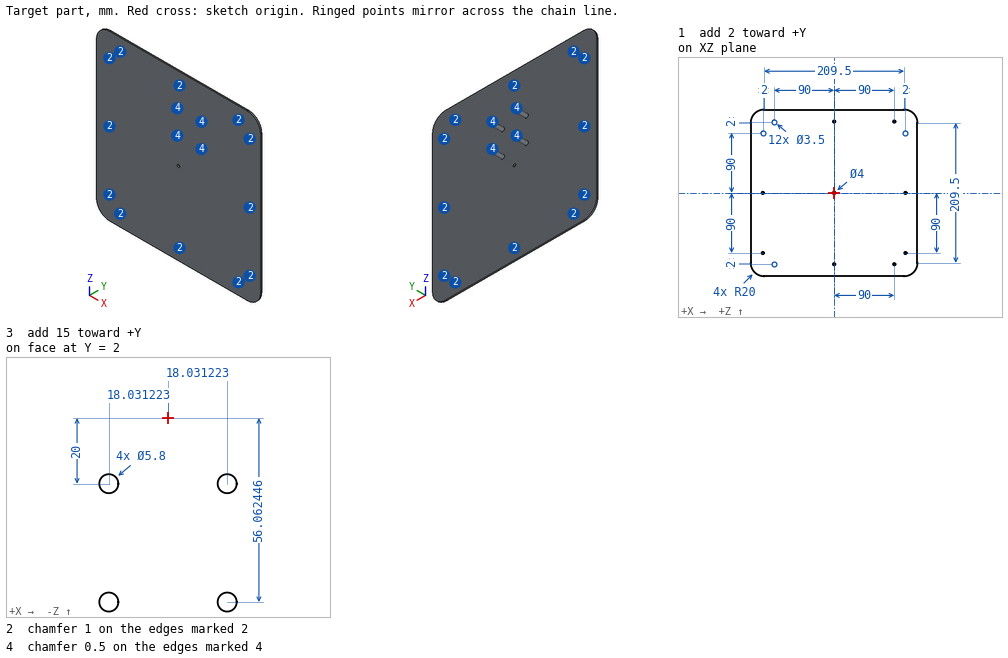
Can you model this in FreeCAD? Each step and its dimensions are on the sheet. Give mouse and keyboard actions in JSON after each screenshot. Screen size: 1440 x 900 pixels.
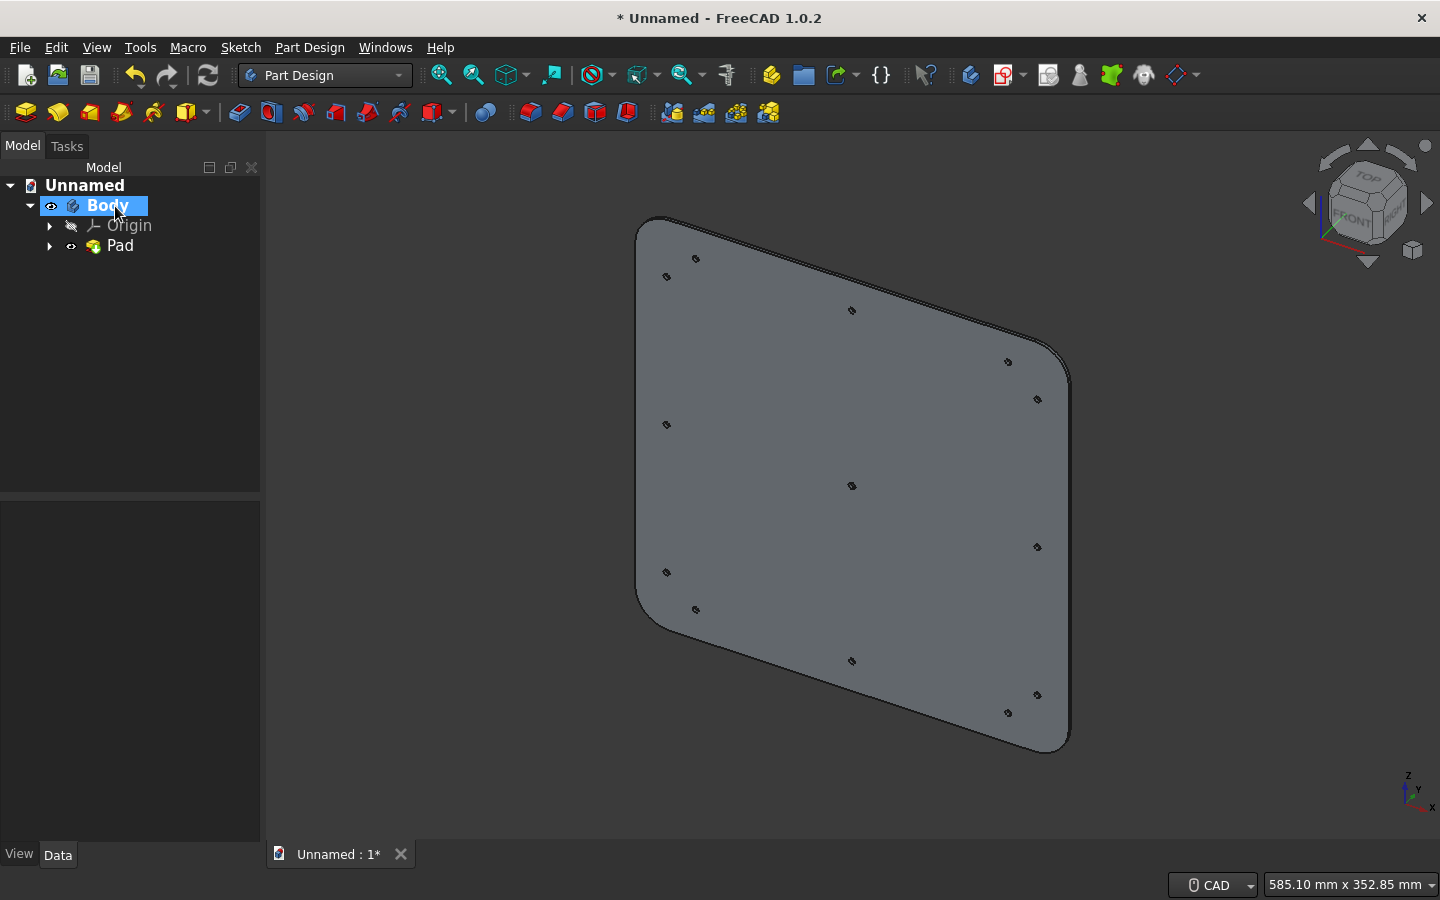
{"action": "key", "text": "0"}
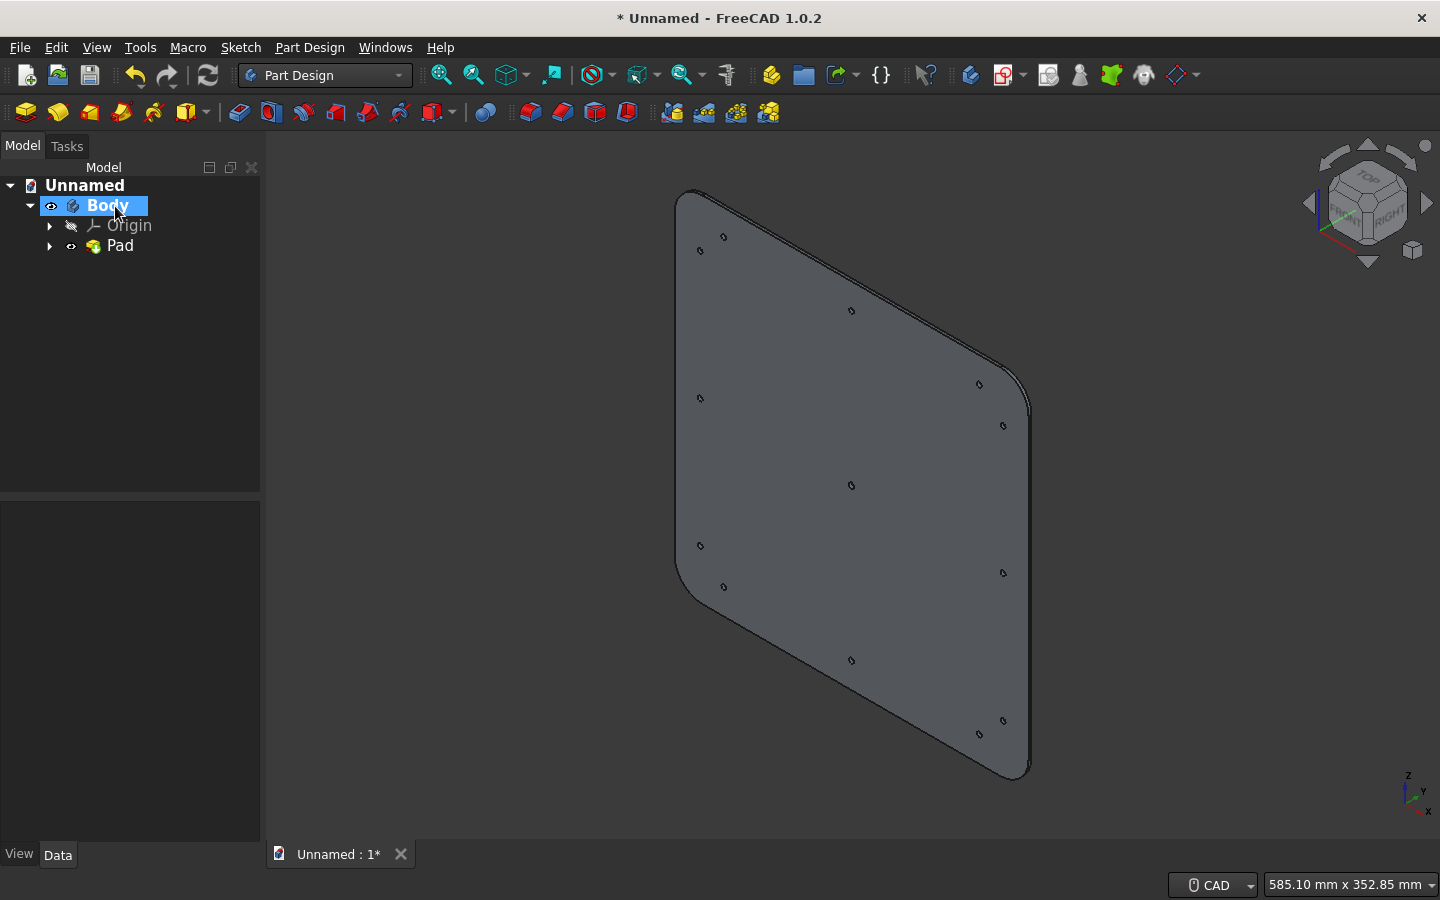
{"action": "key", "text": "2"}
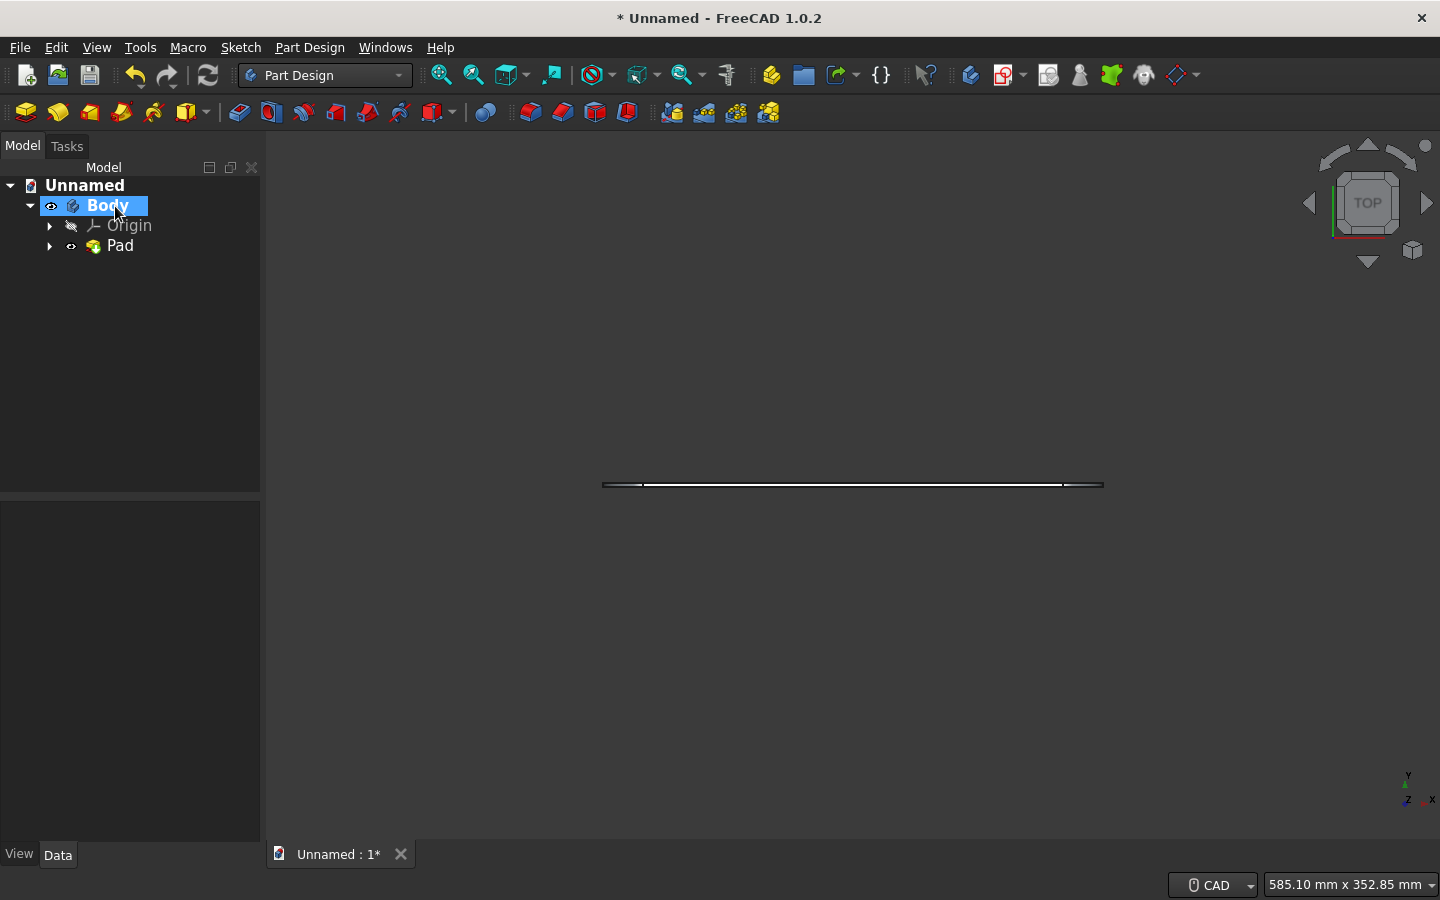
{"action": "key", "text": "v f"}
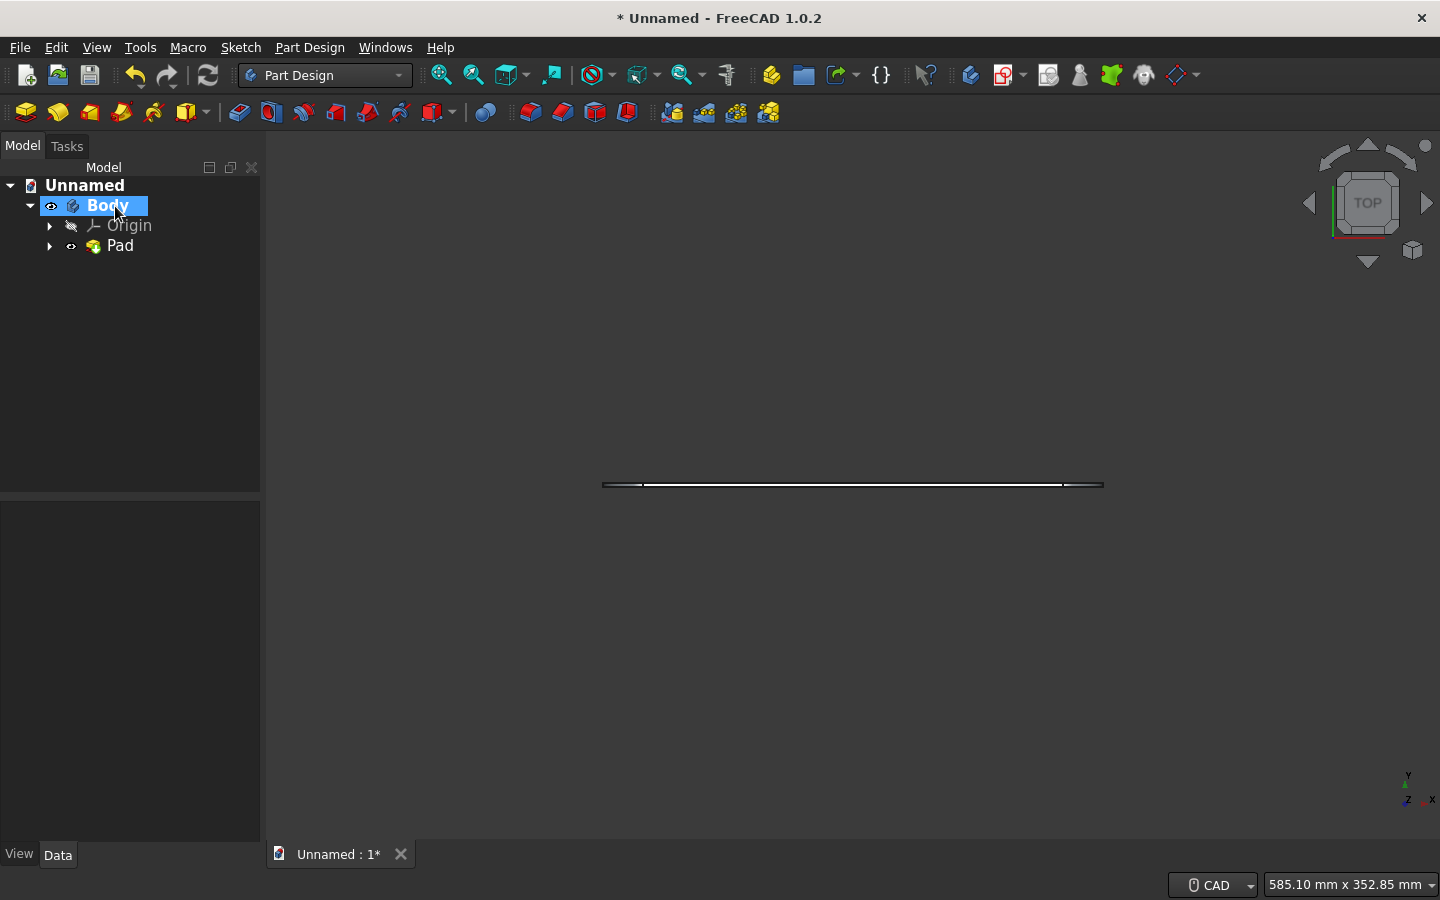
{"action": "key", "text": "1"}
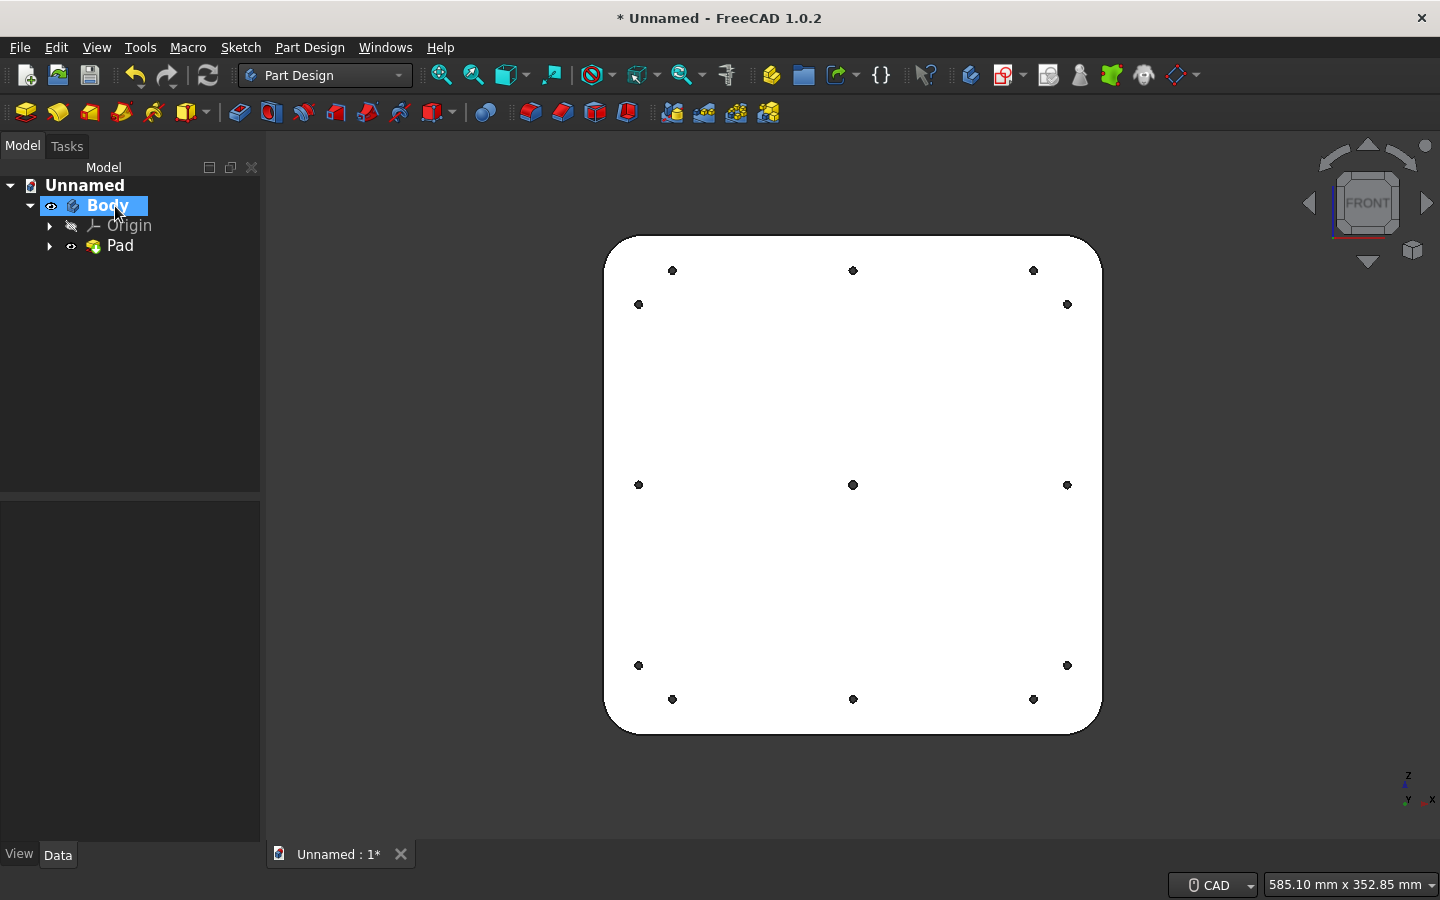
{"action": "key", "text": "3"}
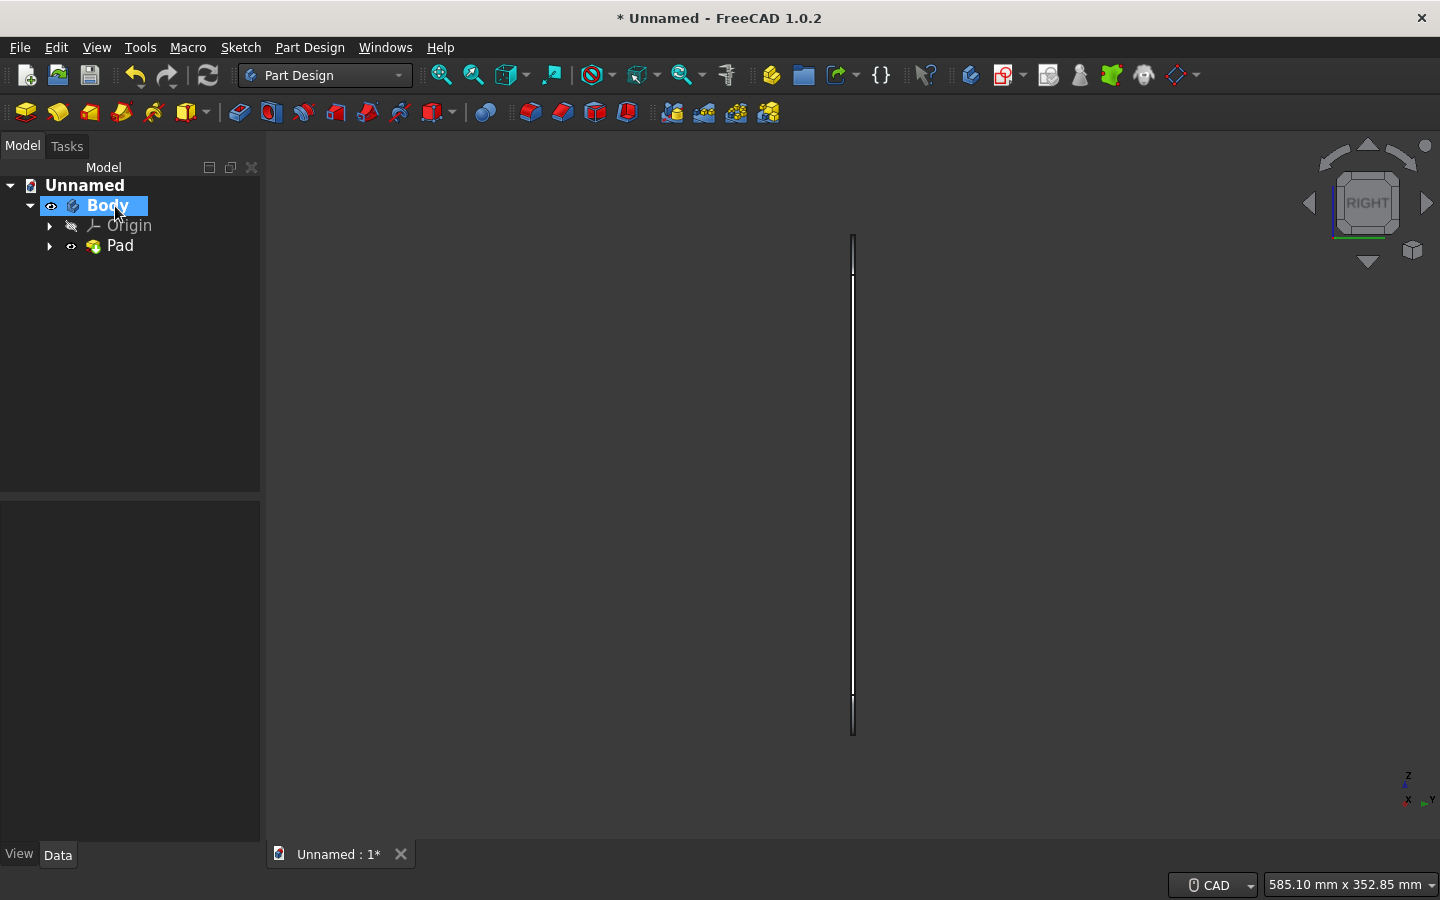
{"action": "key", "text": "5"}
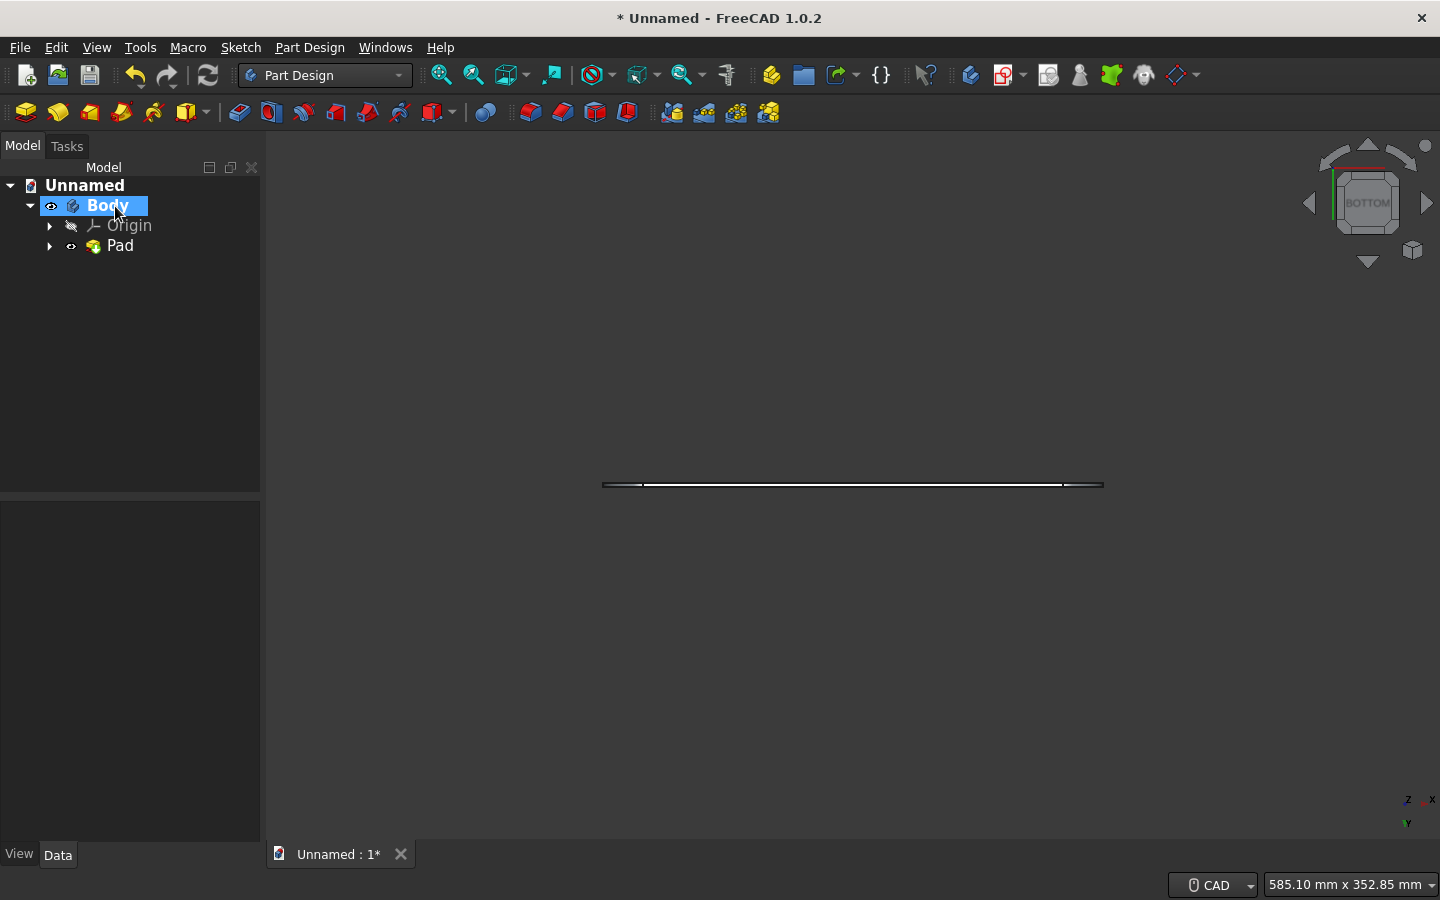
{"action": "key", "text": "v f"}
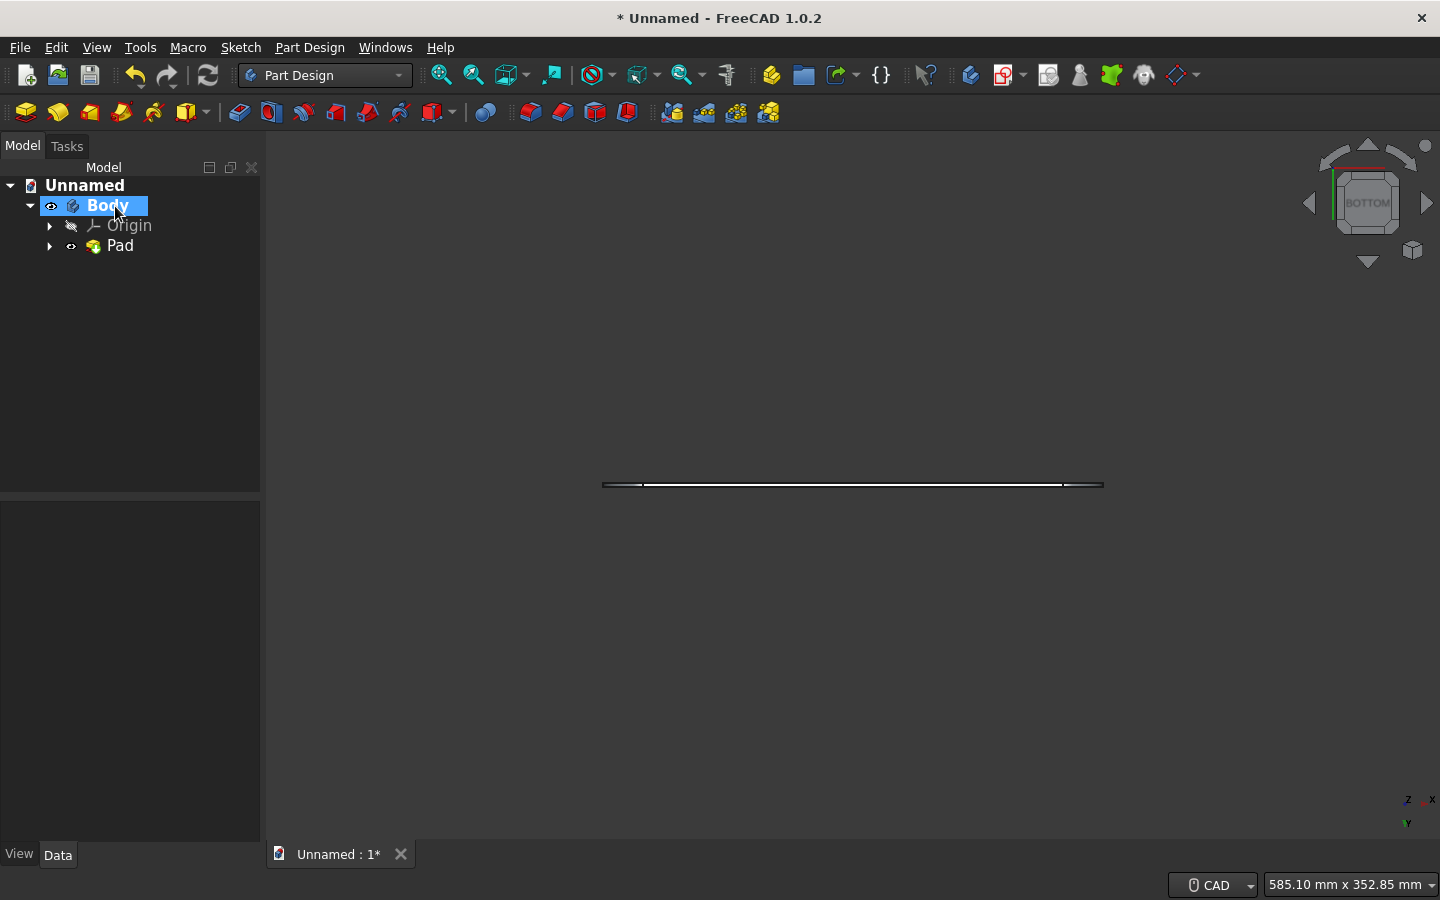
{"action": "key", "text": "4"}